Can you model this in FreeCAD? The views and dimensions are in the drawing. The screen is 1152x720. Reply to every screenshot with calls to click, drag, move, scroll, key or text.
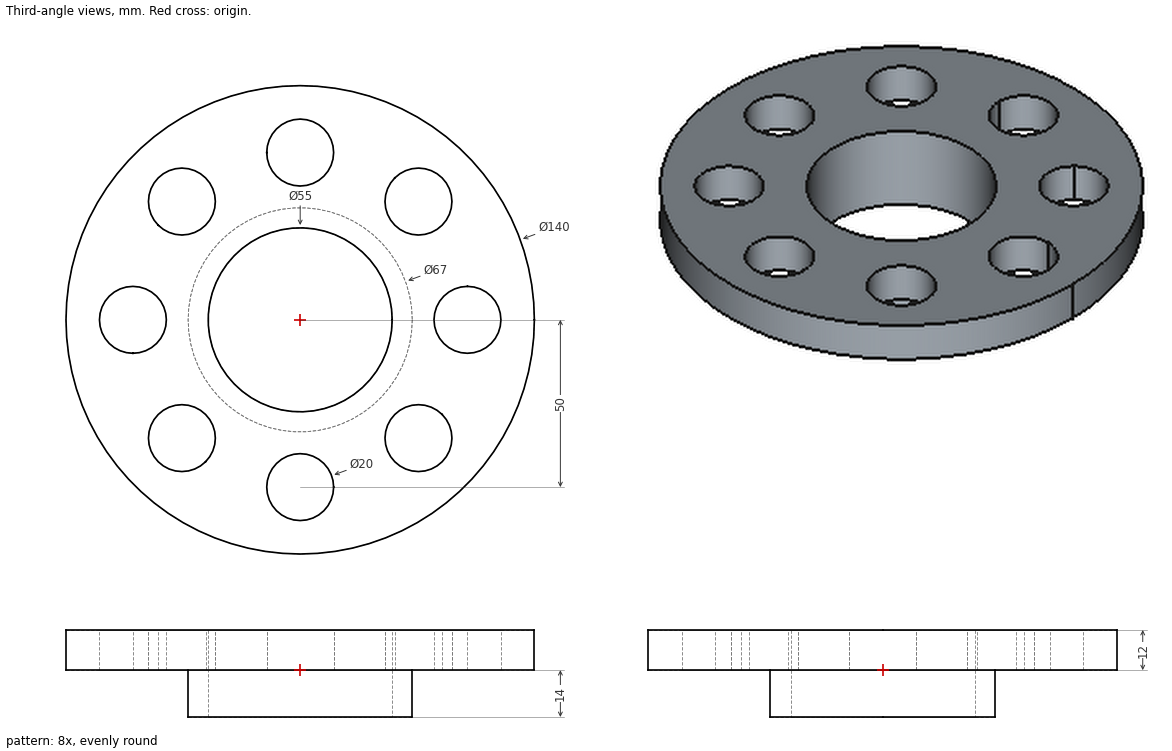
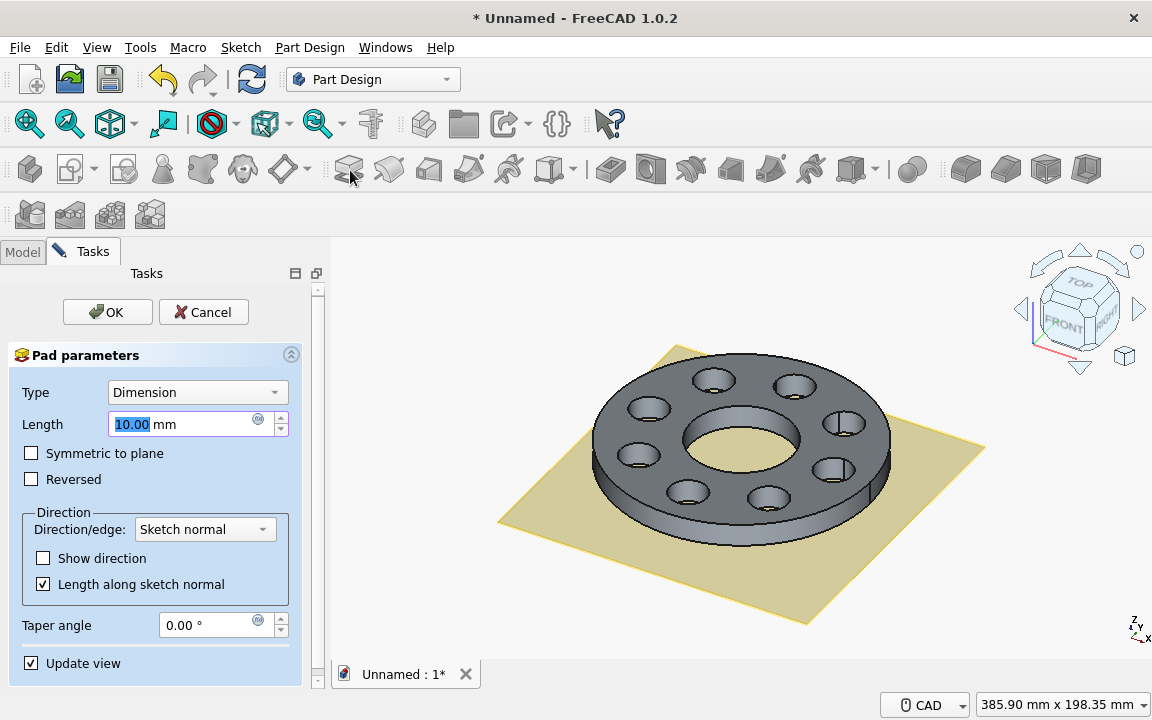
text(14)
key(Tab)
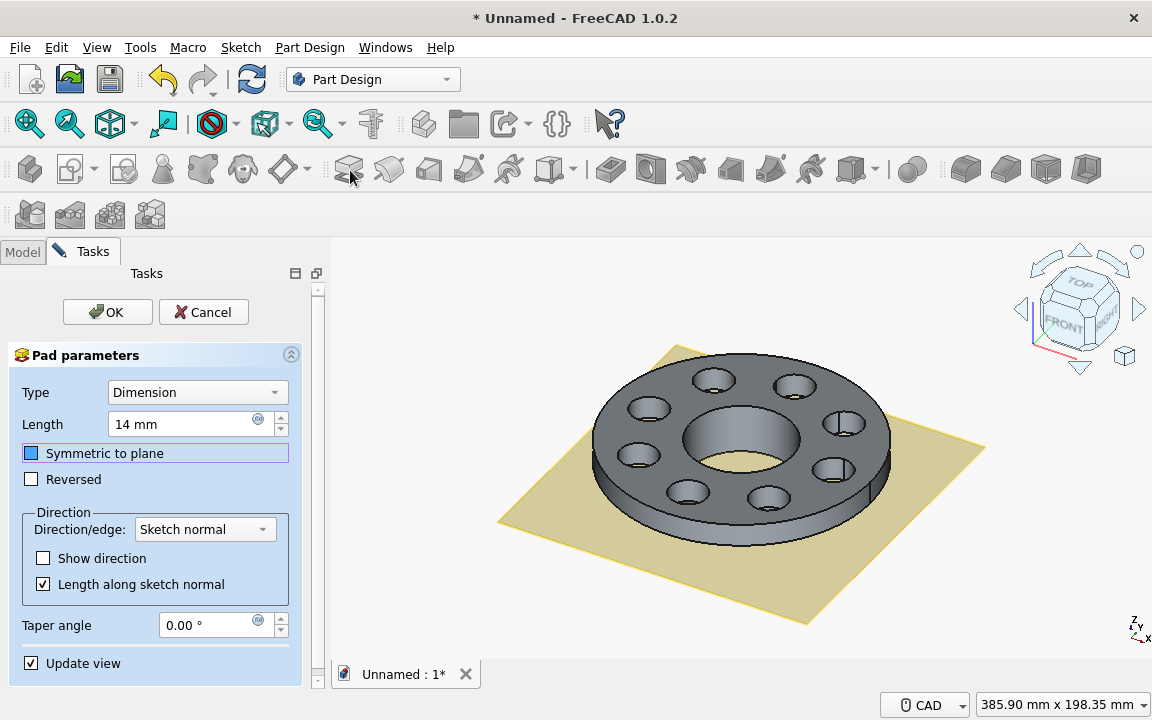
click(108, 312)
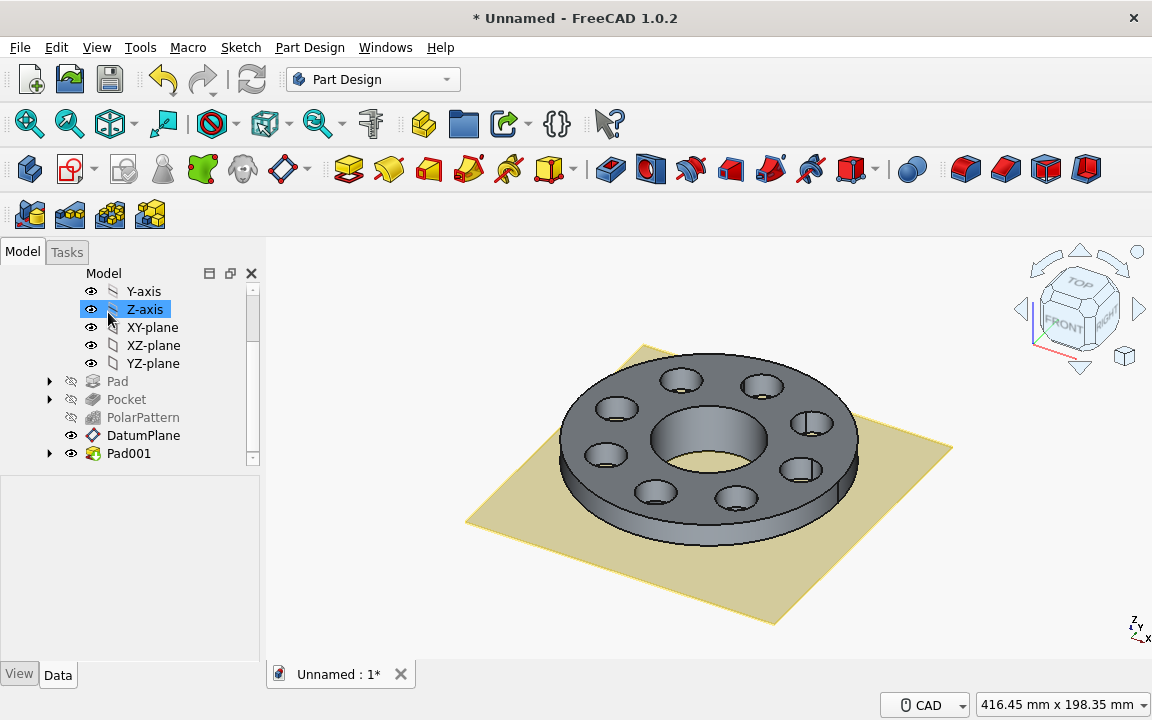
click(116, 435)
key(space)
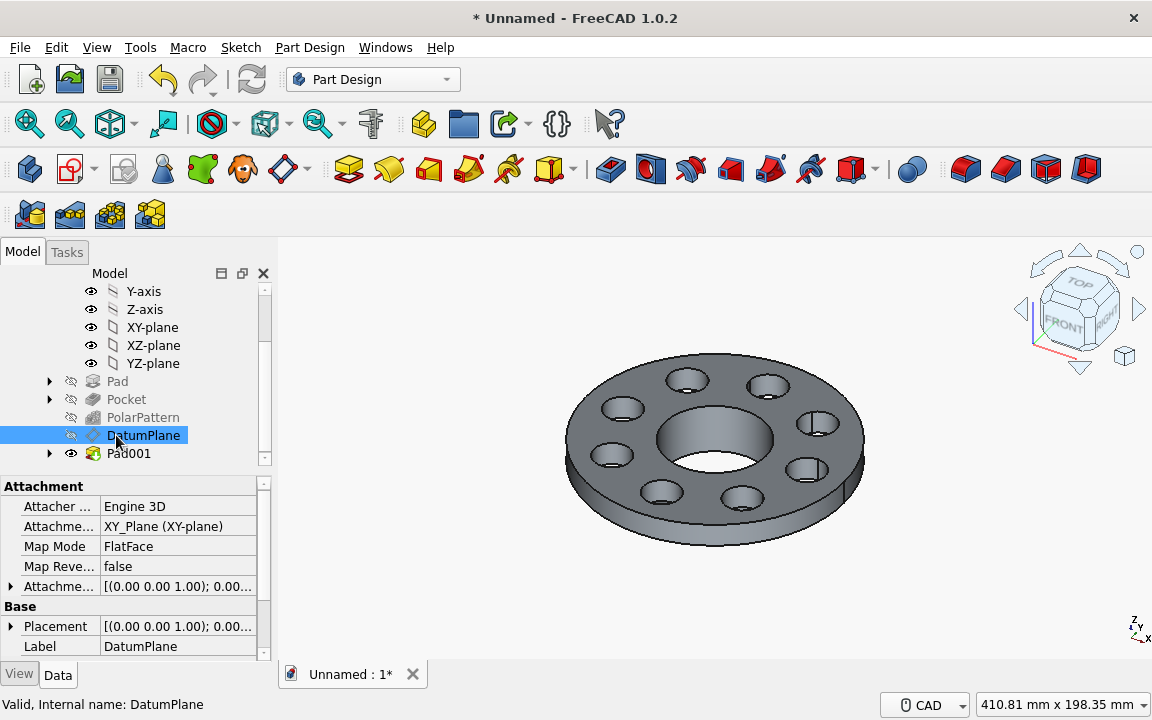
key(0)